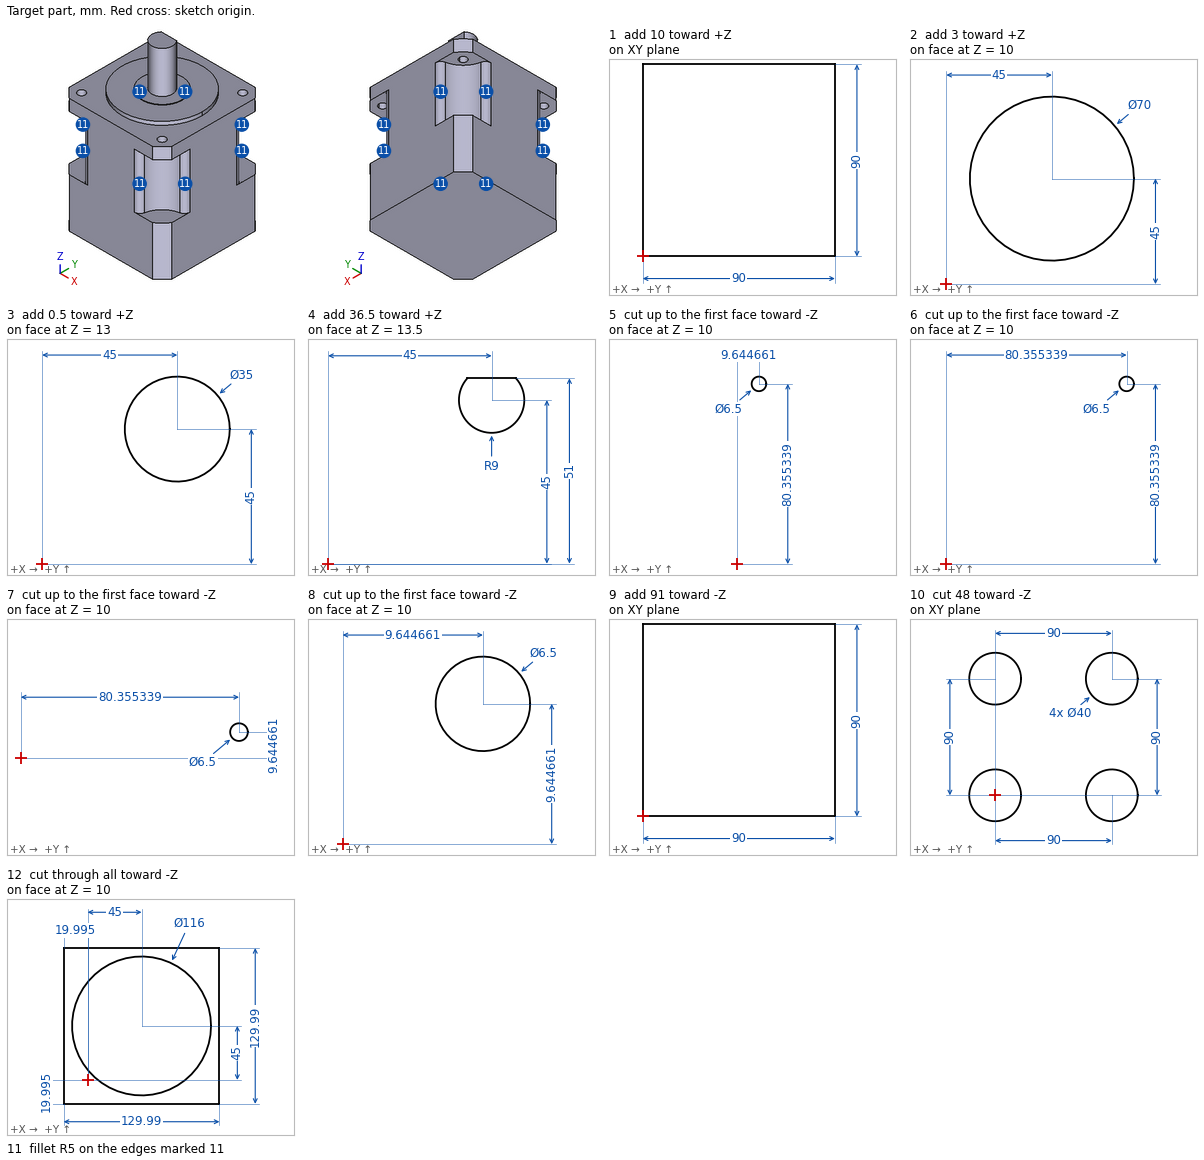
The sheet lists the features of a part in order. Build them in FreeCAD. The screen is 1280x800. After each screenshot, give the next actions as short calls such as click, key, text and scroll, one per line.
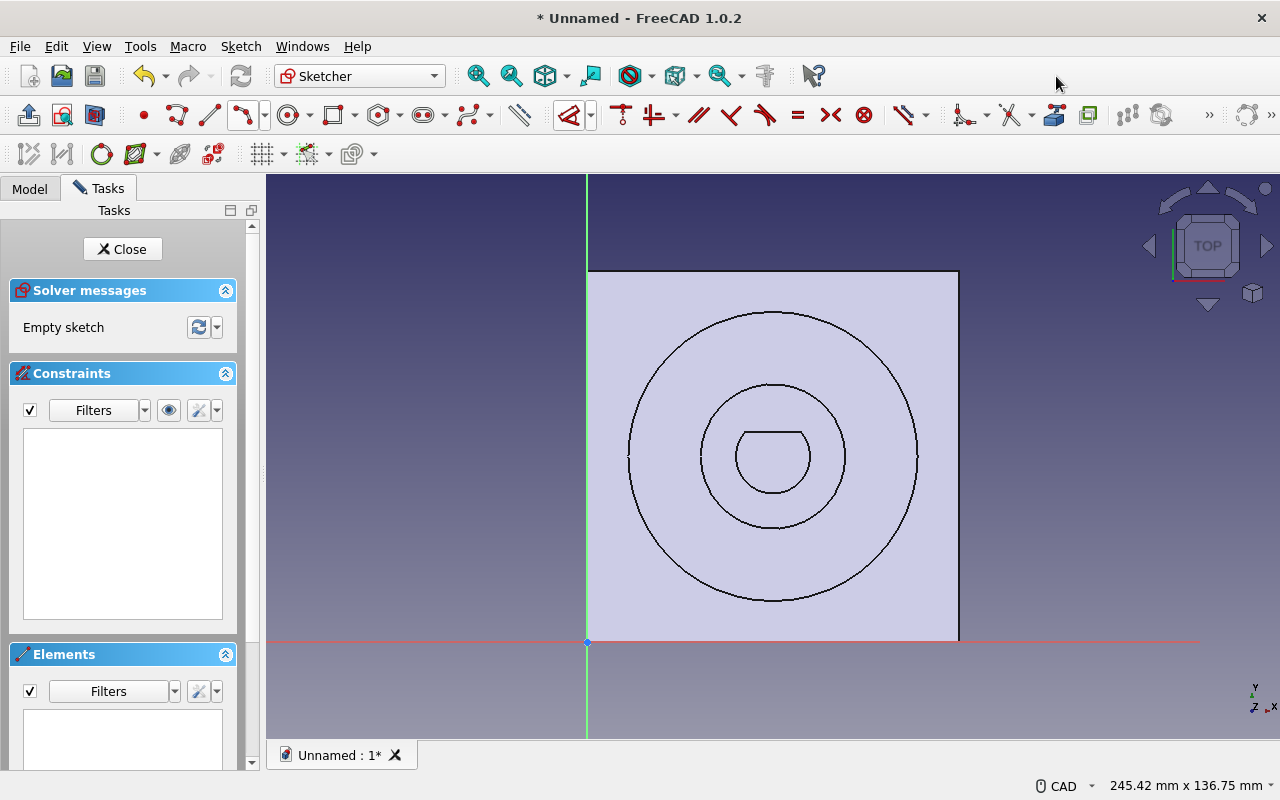
scroll(621, 299, up, 13)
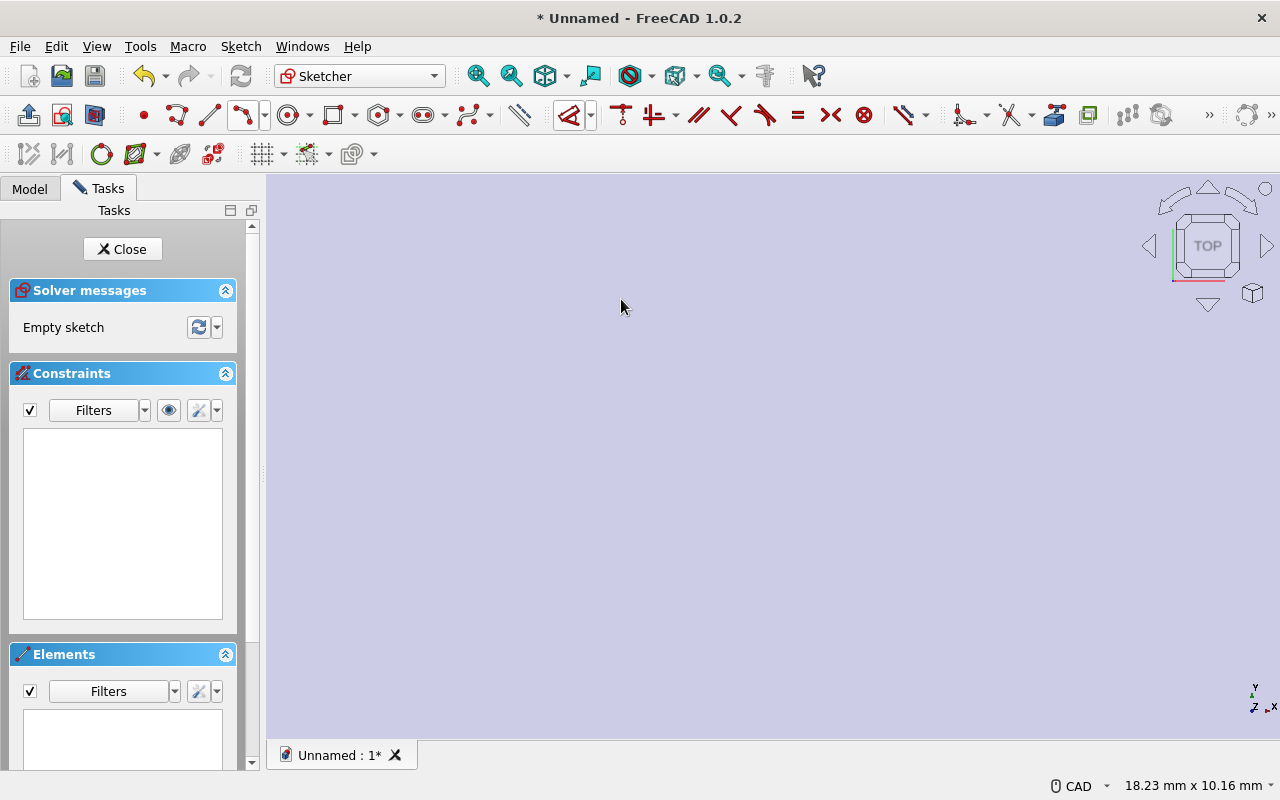
click(288, 116)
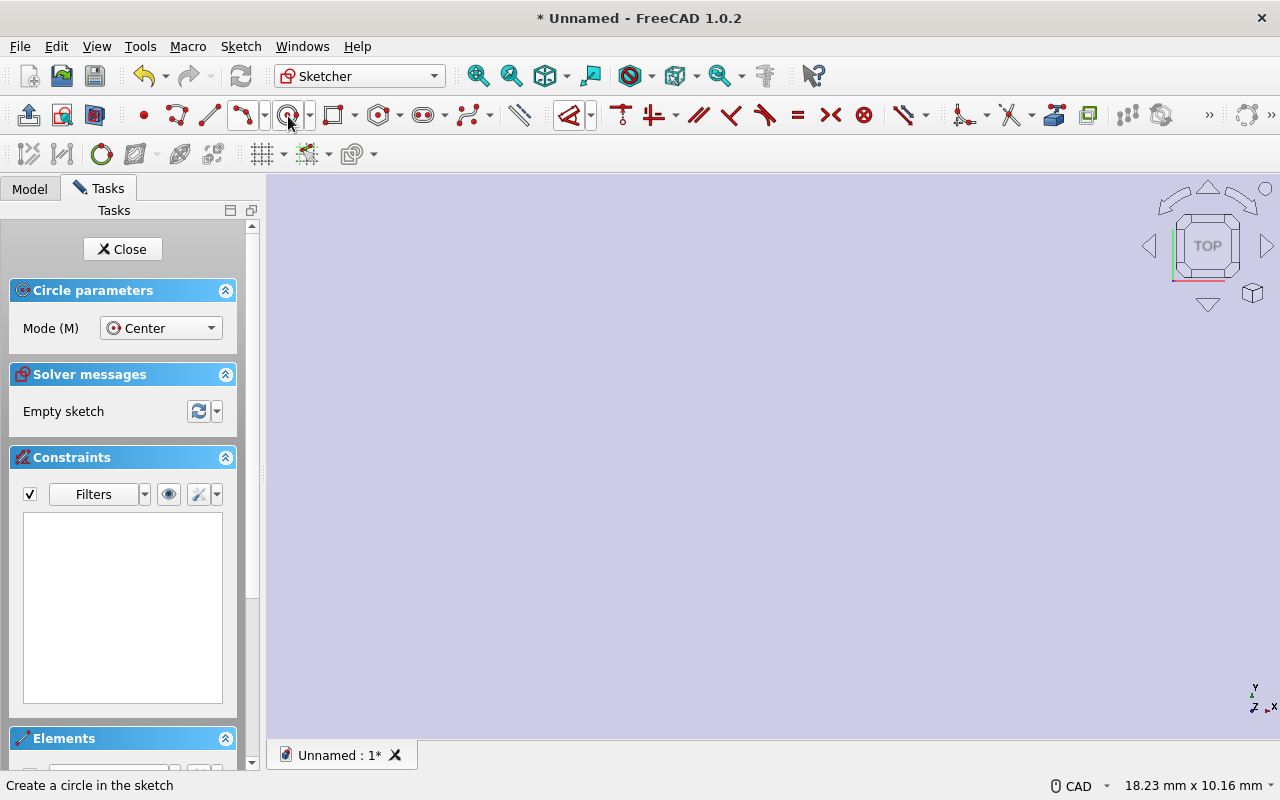
click(696, 450)
move(824, 322)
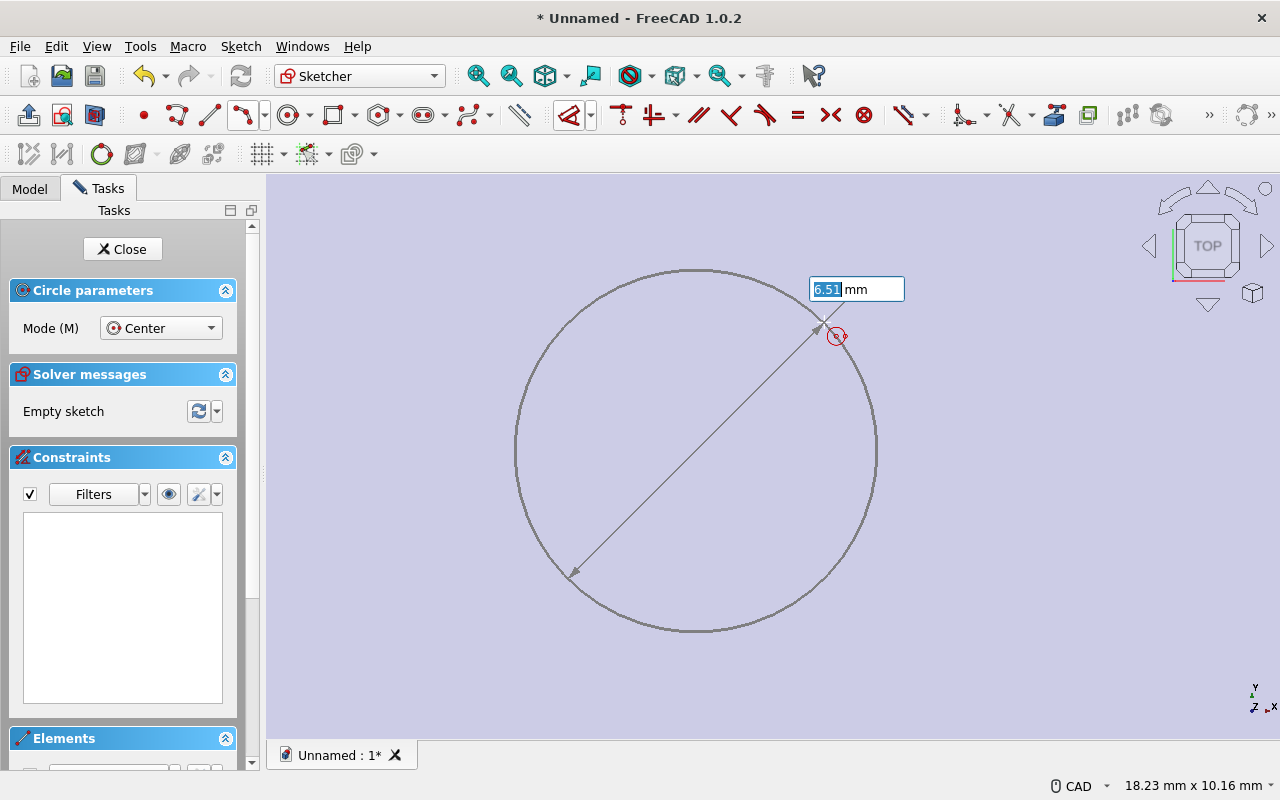
text(6.5)
key(Return)
key(Escape)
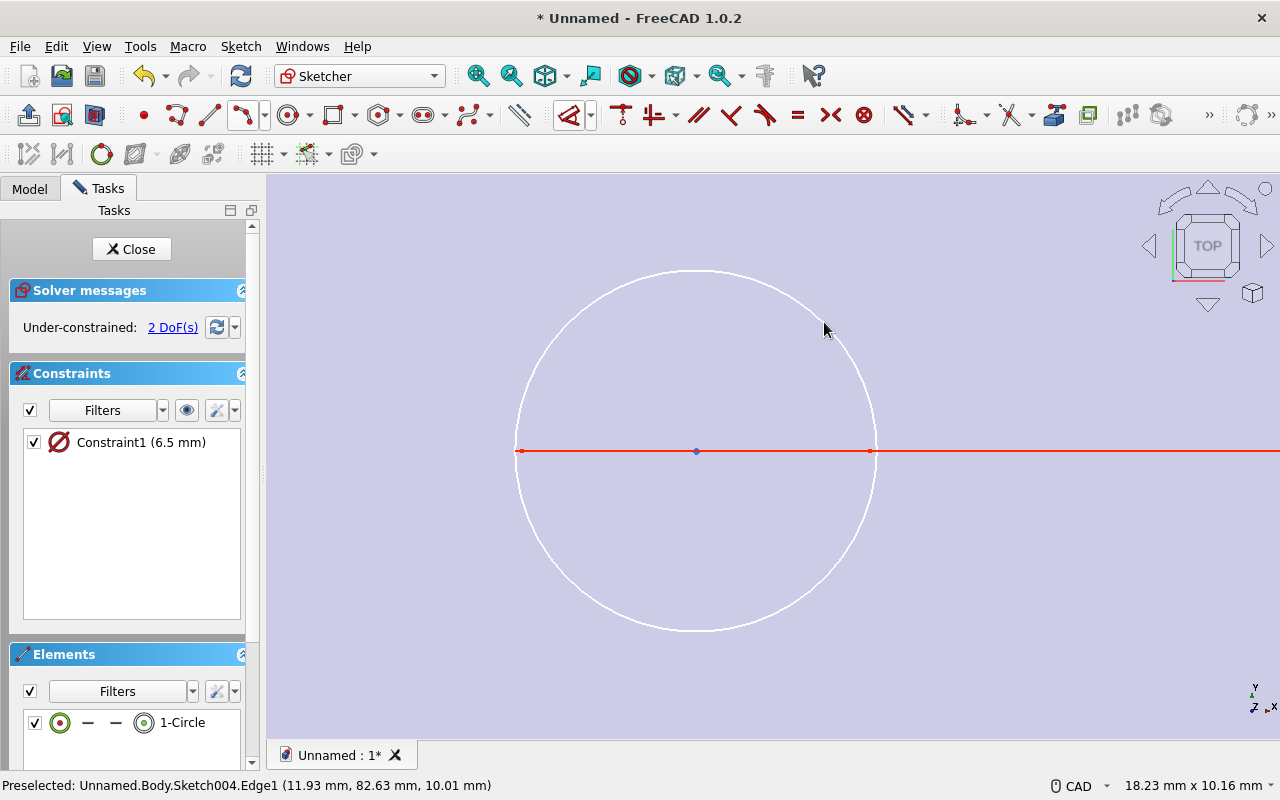
click(696, 451)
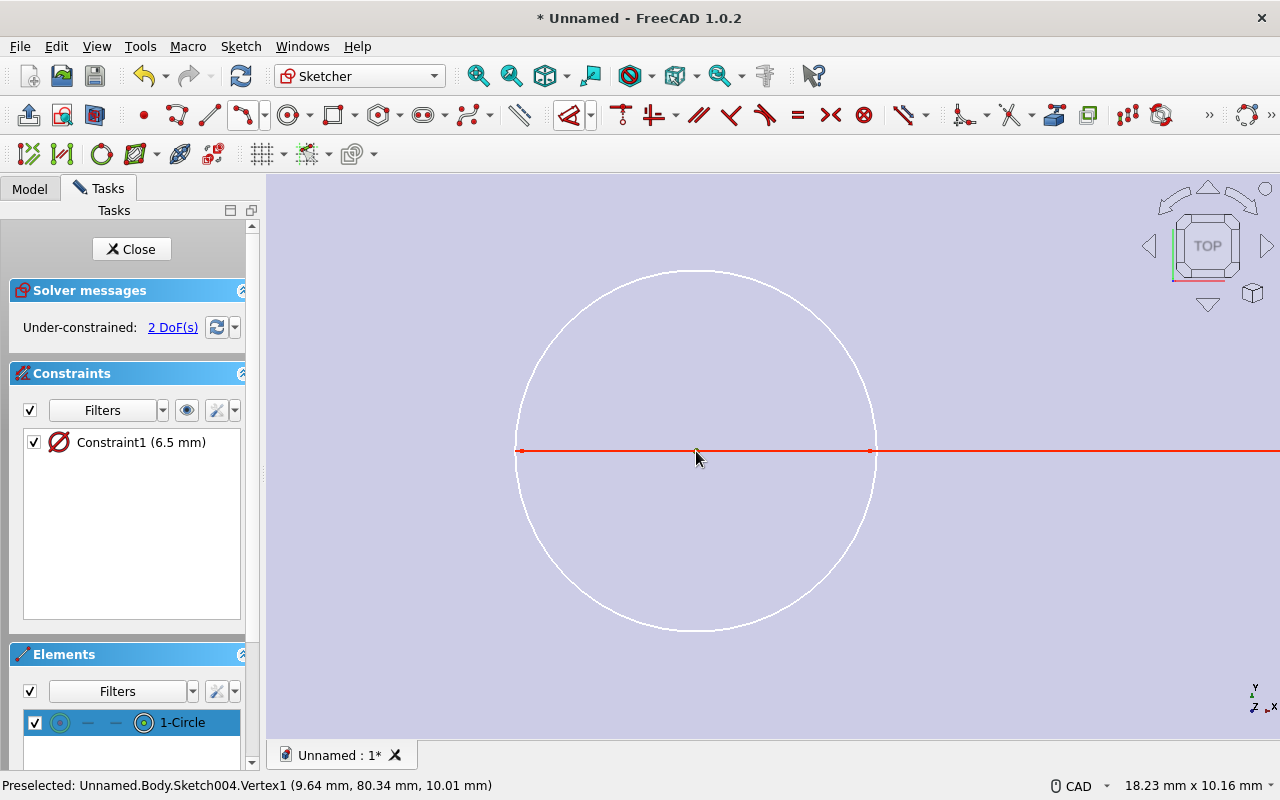
click(590, 116)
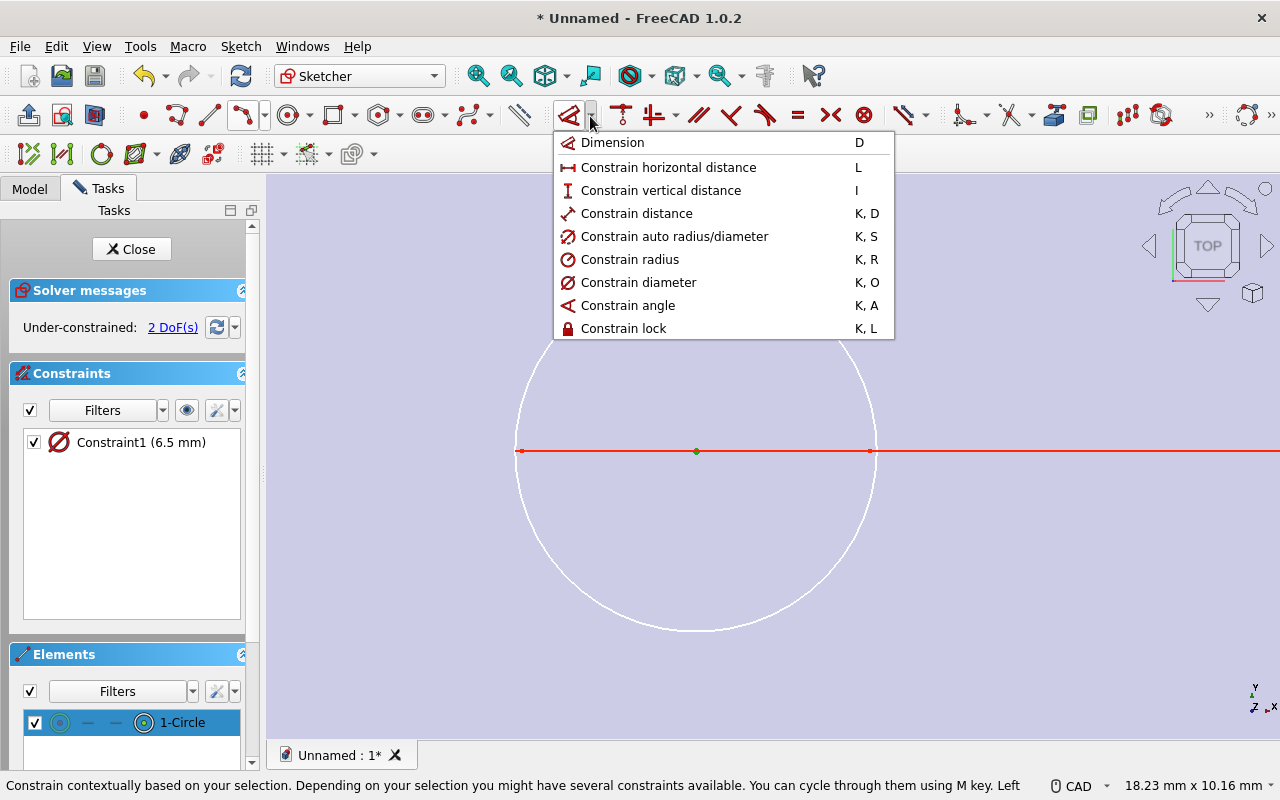
click(724, 168)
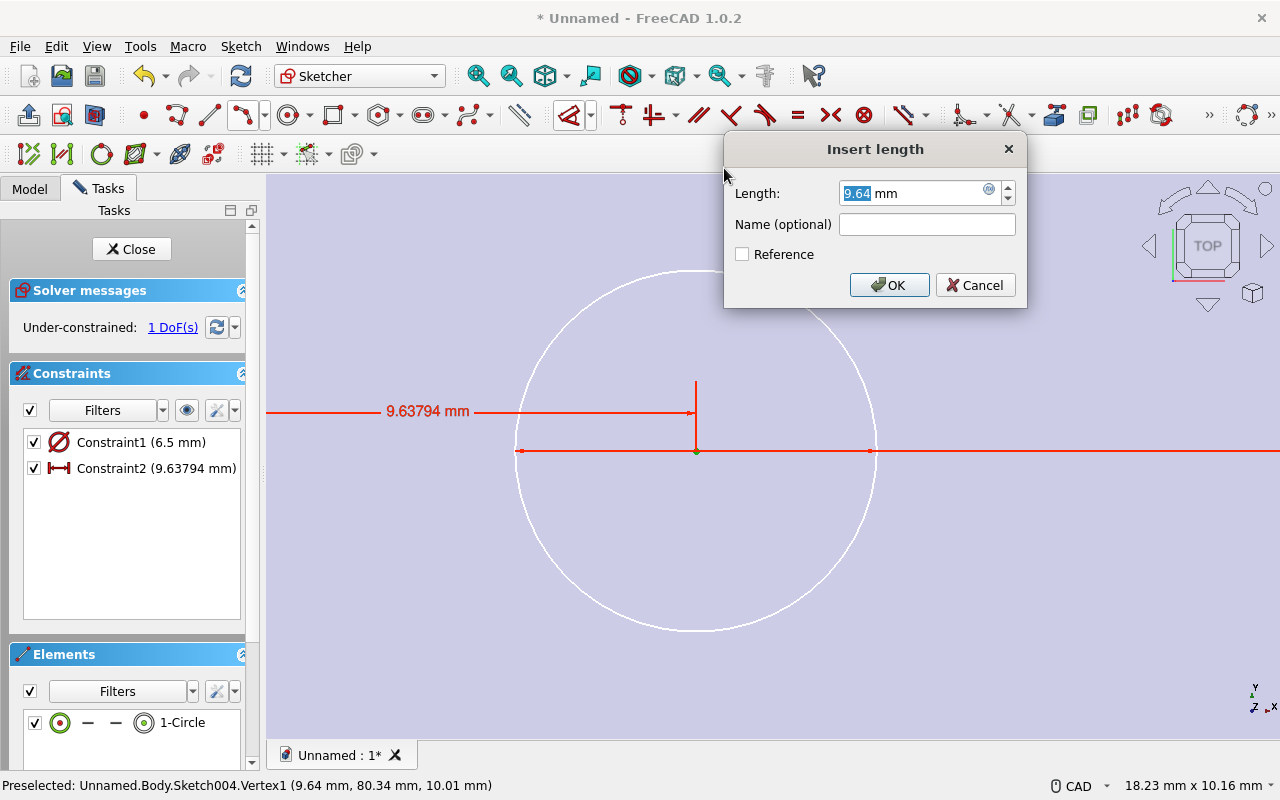
text(9.644661)
key(Return)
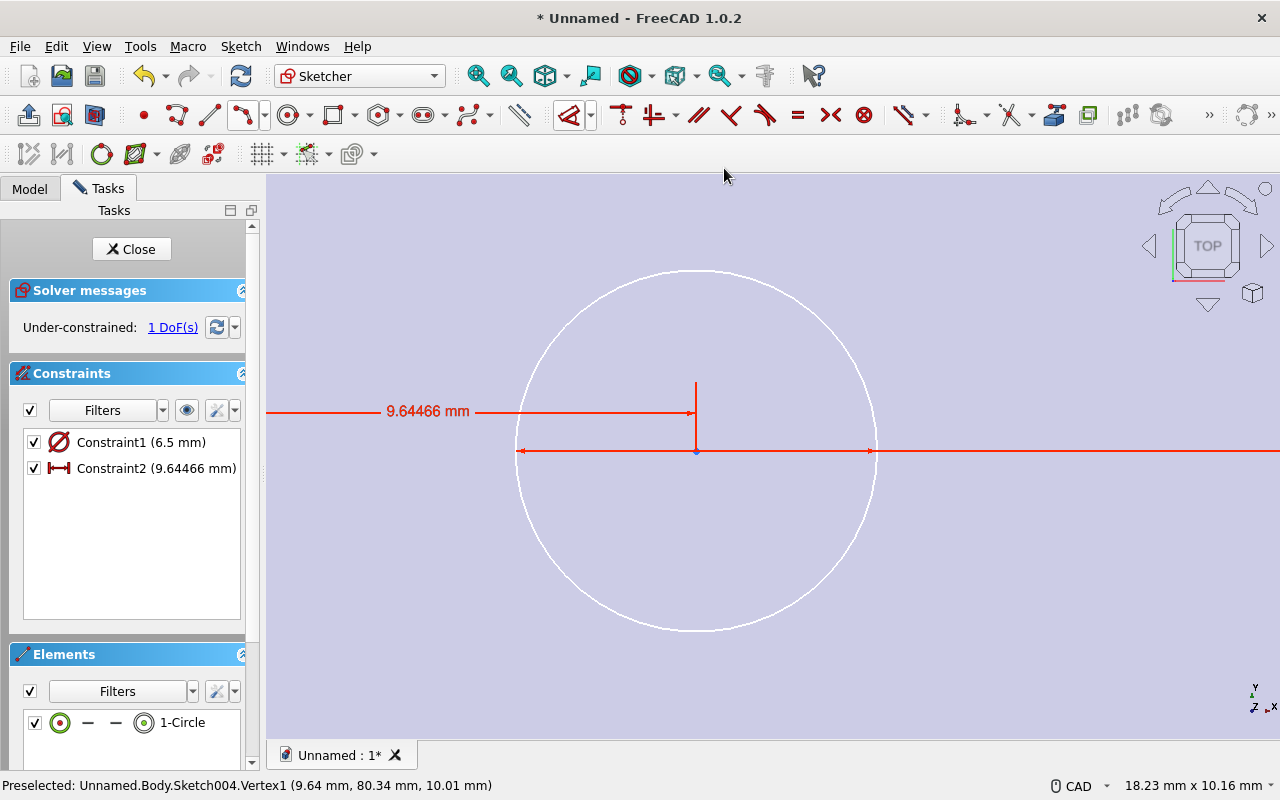
click(696, 451)